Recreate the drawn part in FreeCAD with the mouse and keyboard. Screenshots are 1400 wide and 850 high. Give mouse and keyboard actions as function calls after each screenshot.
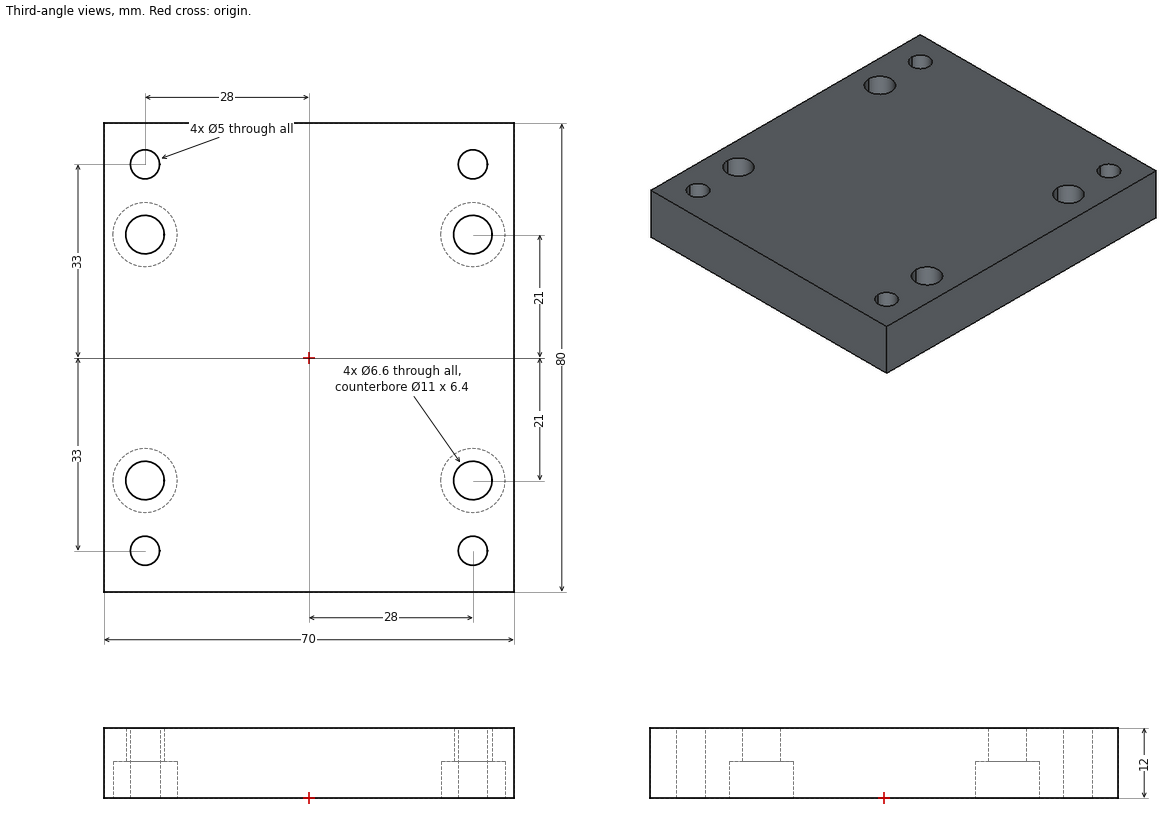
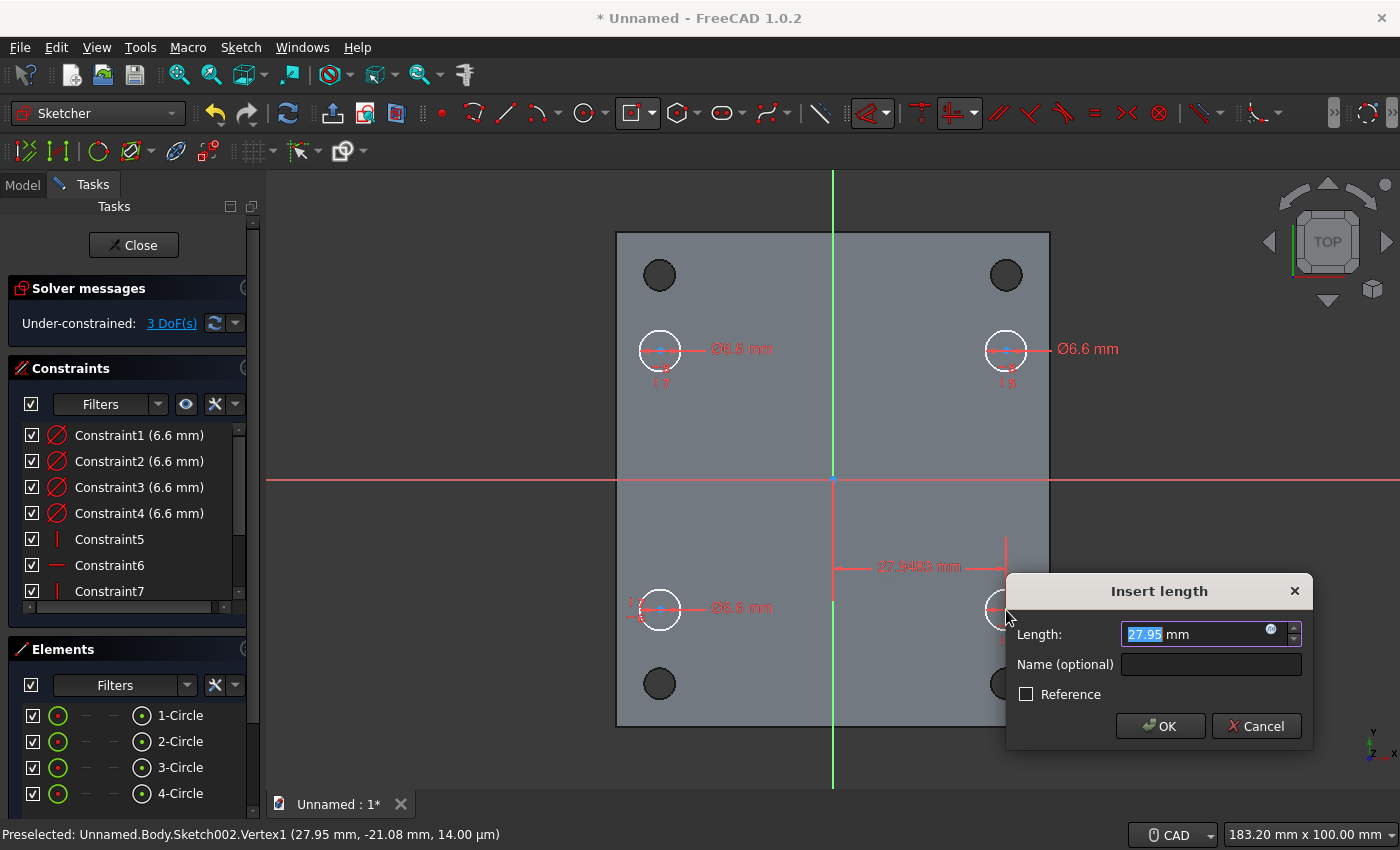
text(28)
key(Return)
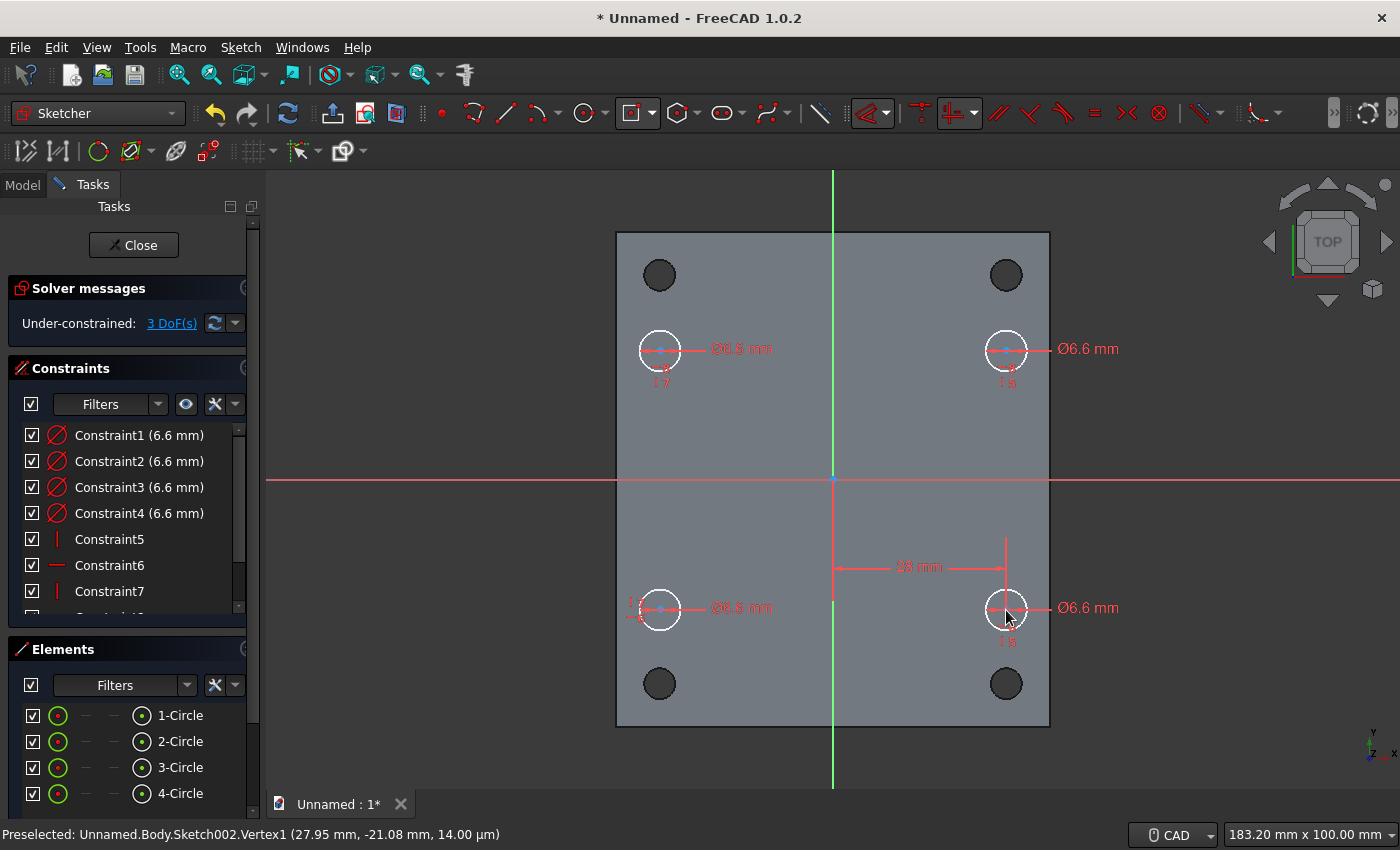
click(1006, 610)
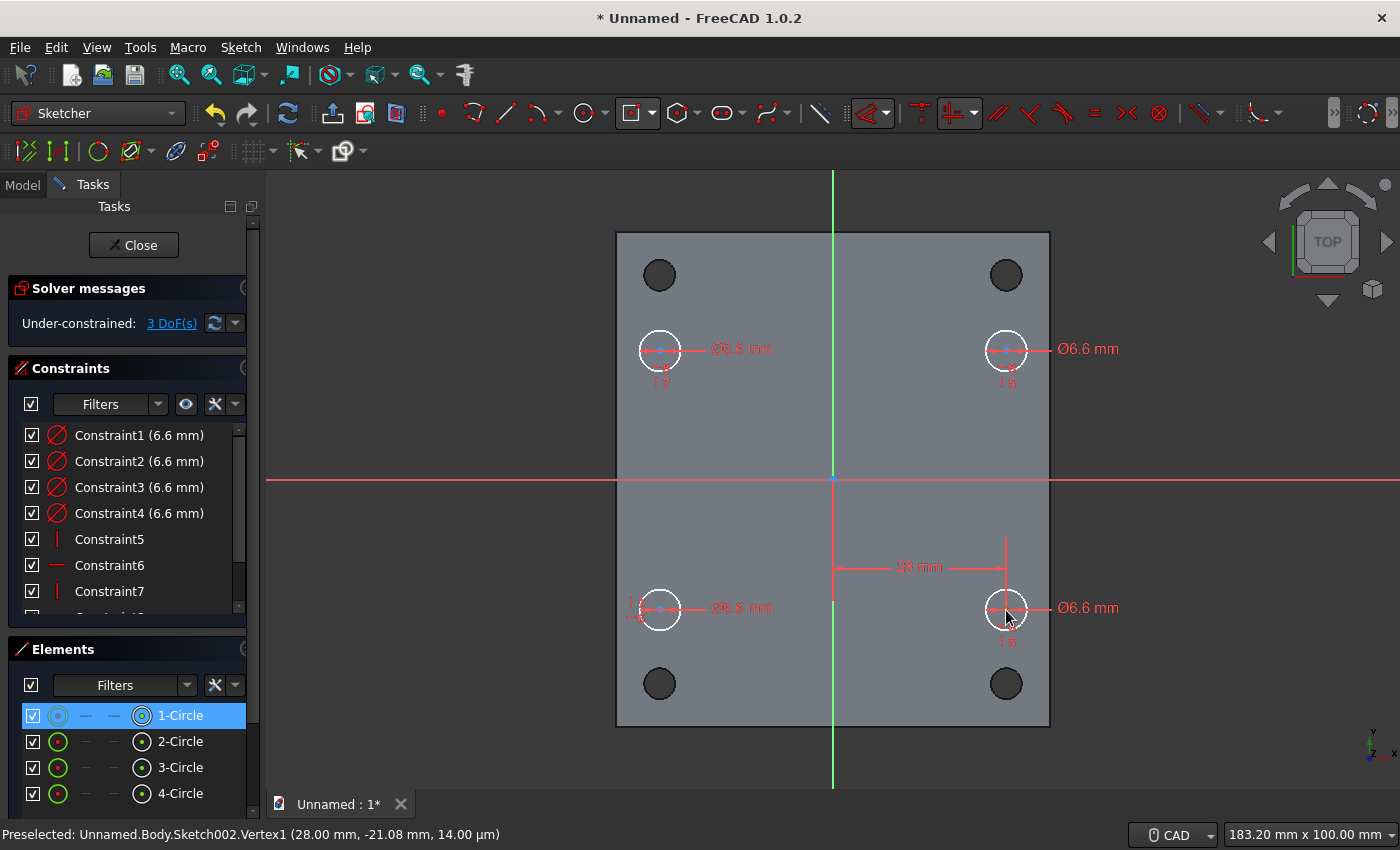
key(i)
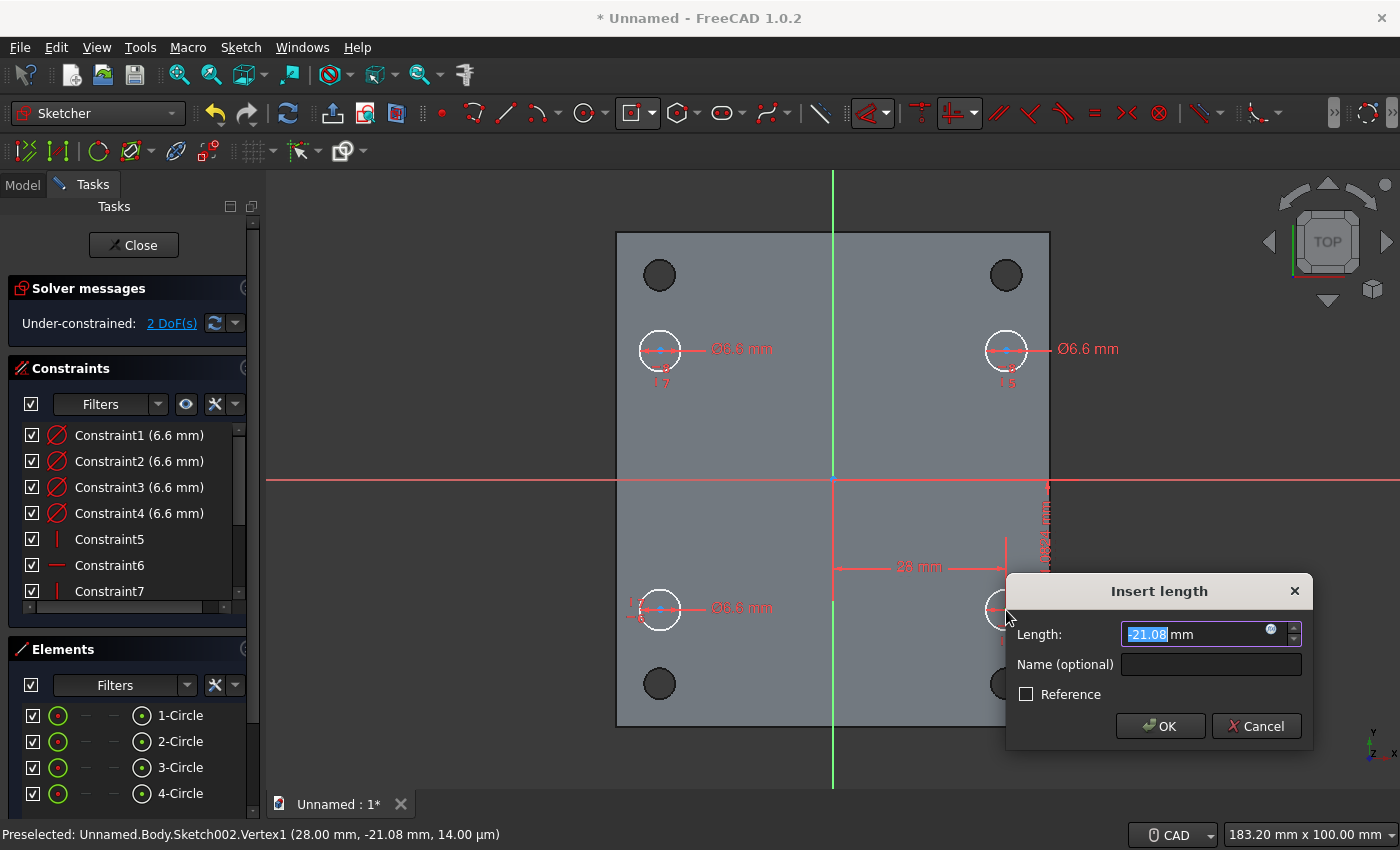
text(-21)
key(Return)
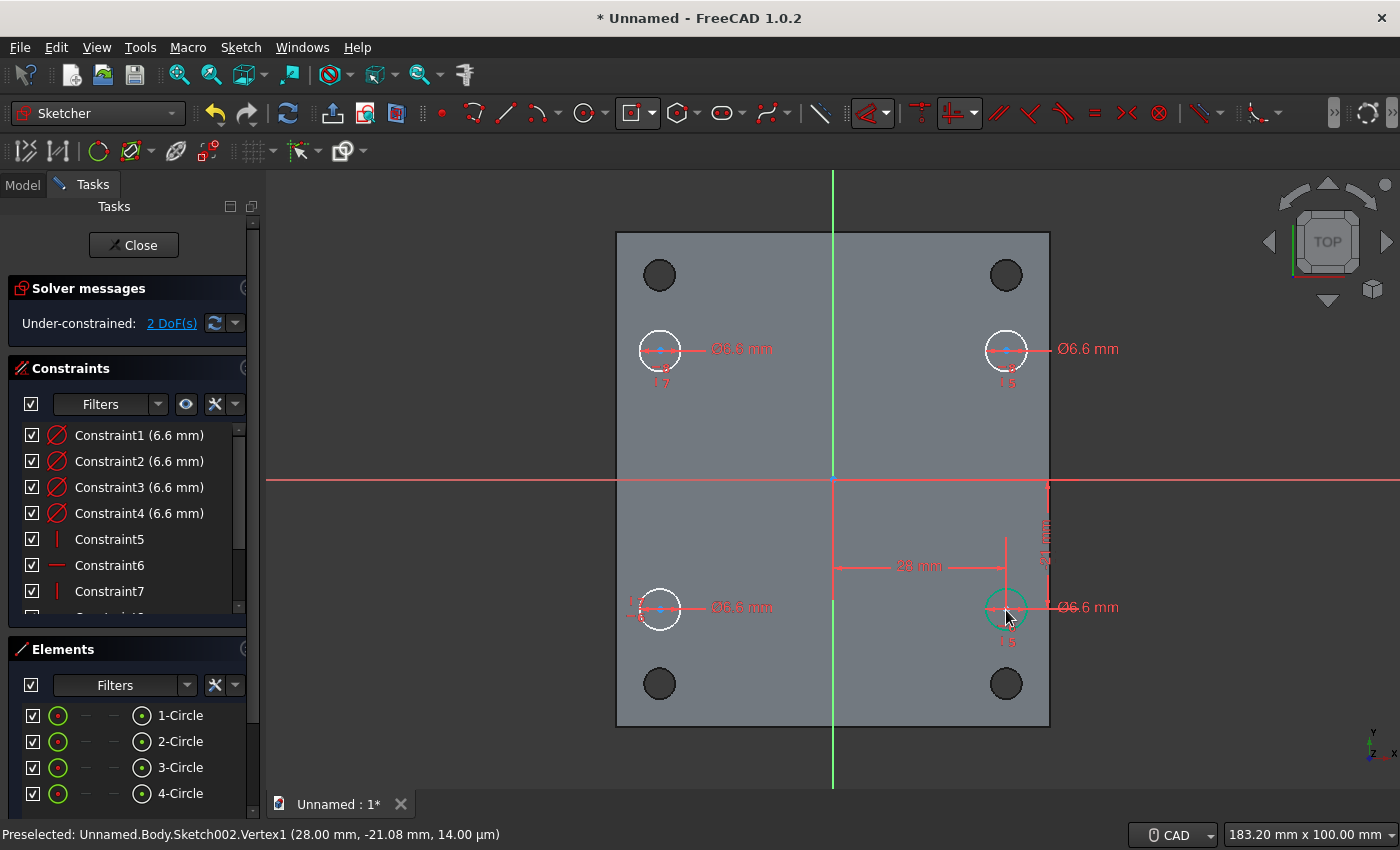
click(1006, 351)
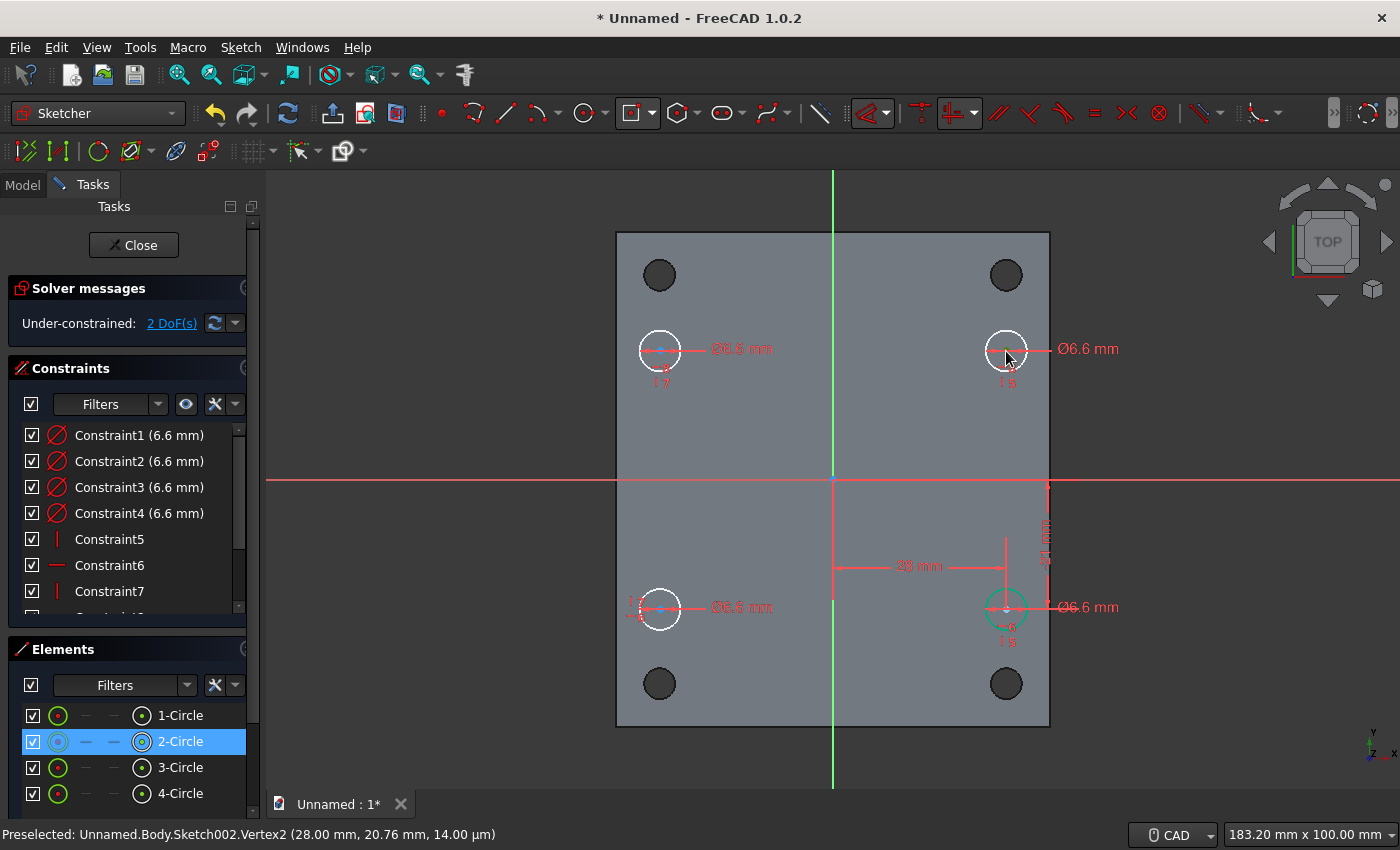
click(888, 114)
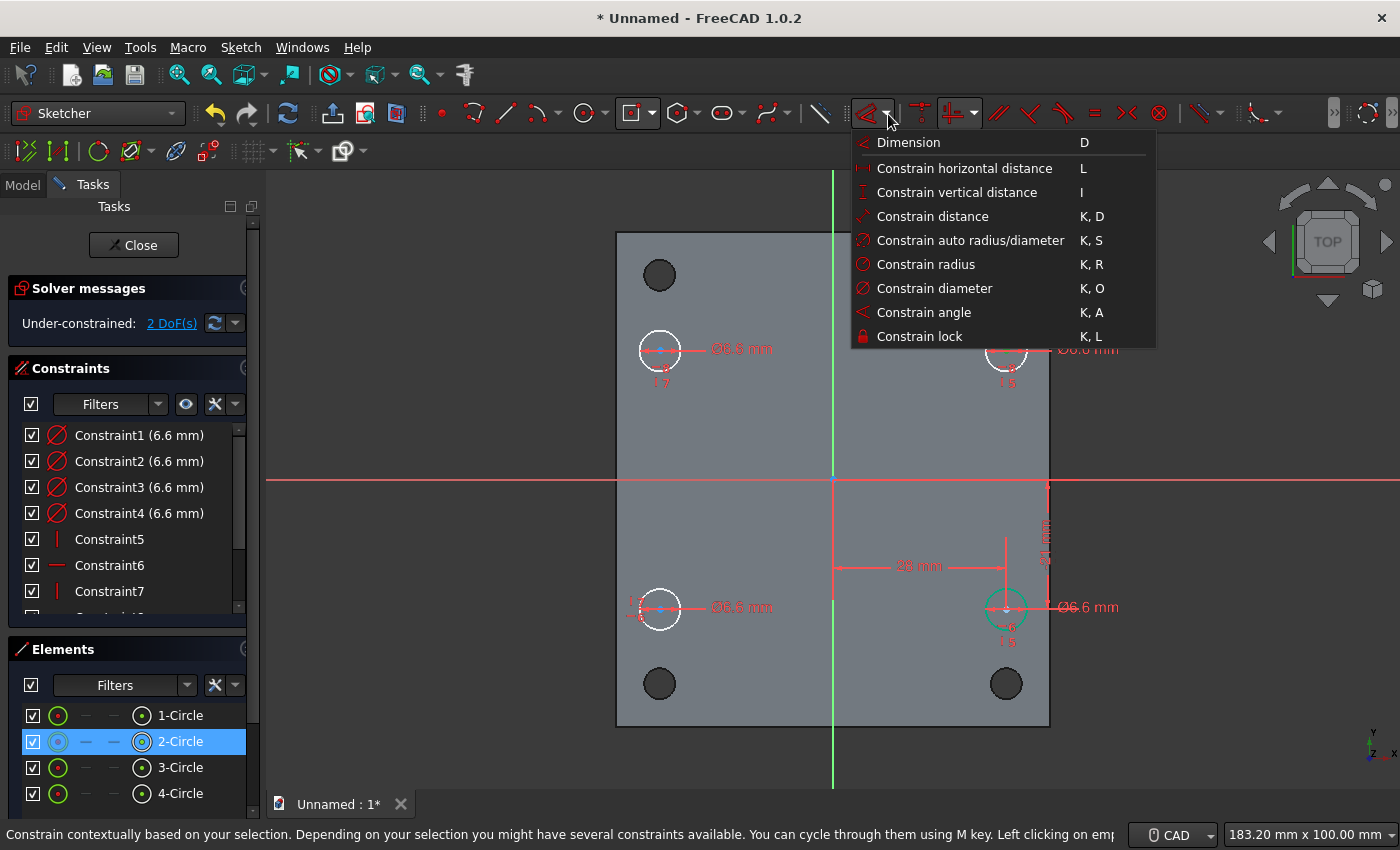
click(1004, 192)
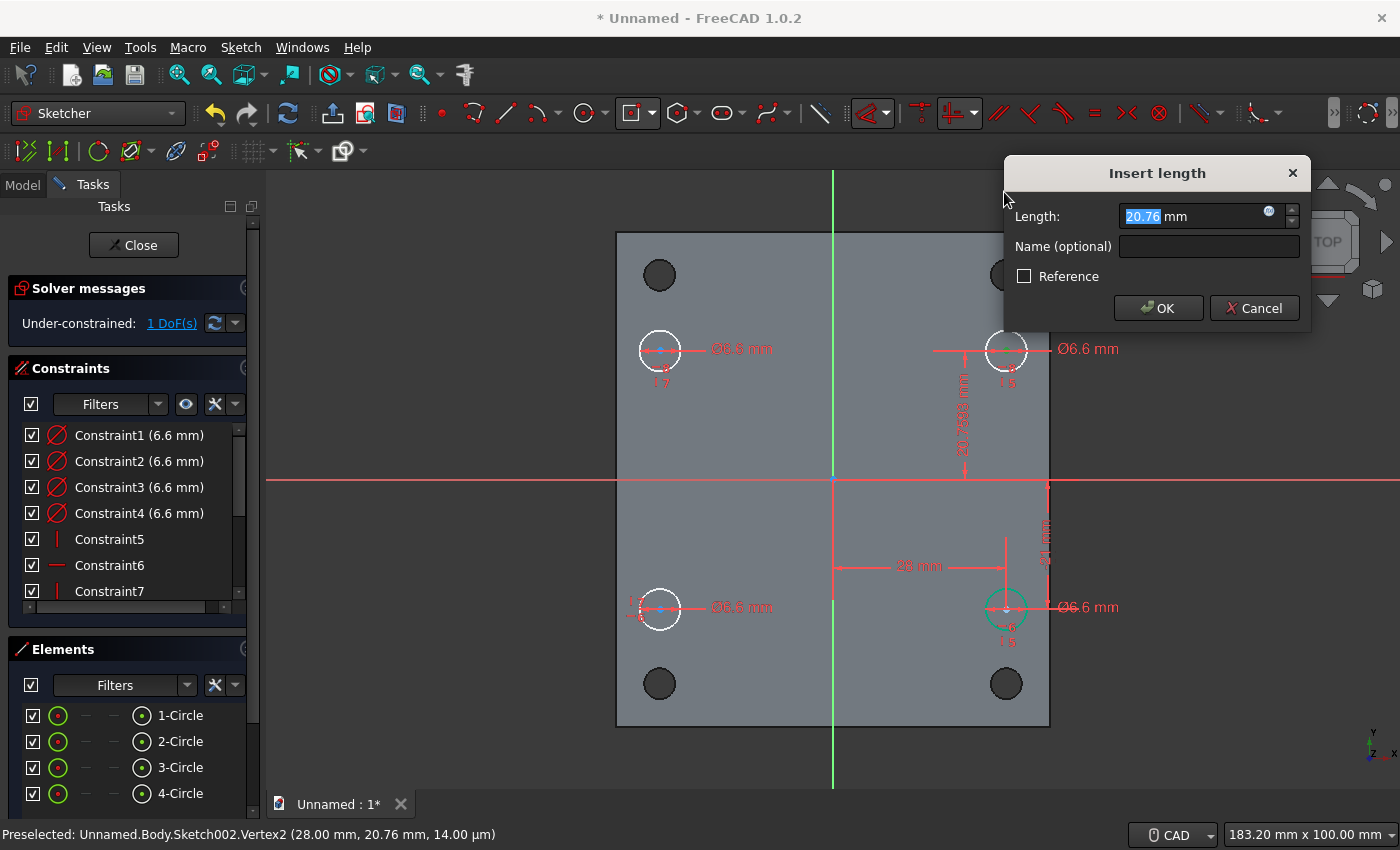
text(21)
key(Return)